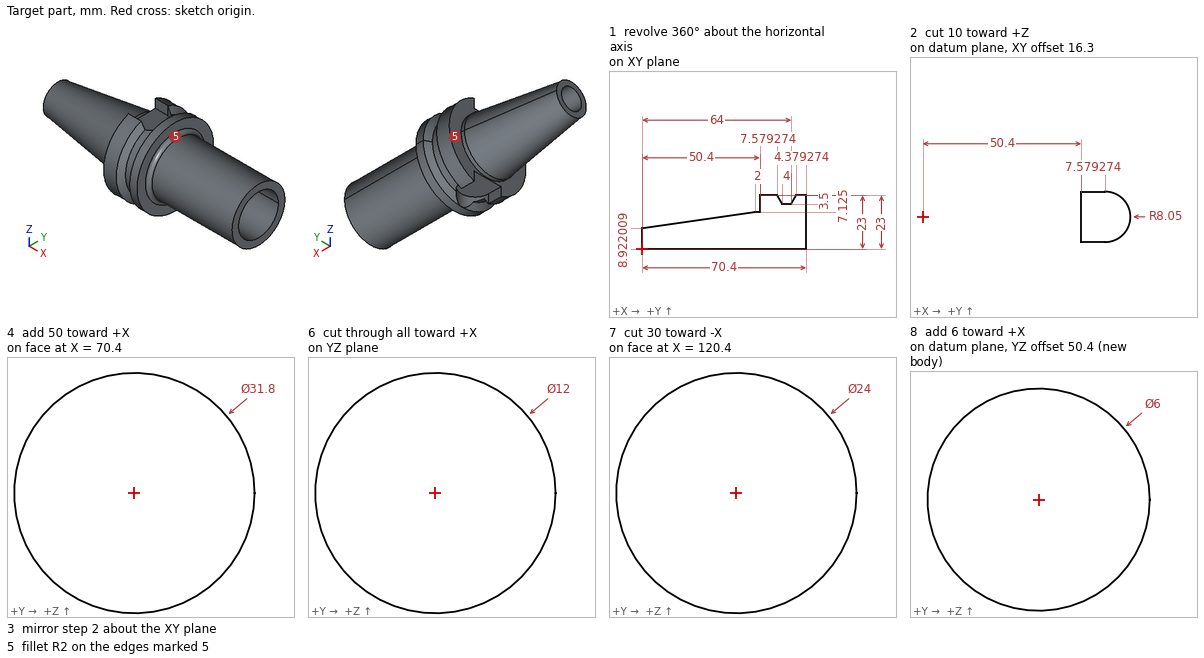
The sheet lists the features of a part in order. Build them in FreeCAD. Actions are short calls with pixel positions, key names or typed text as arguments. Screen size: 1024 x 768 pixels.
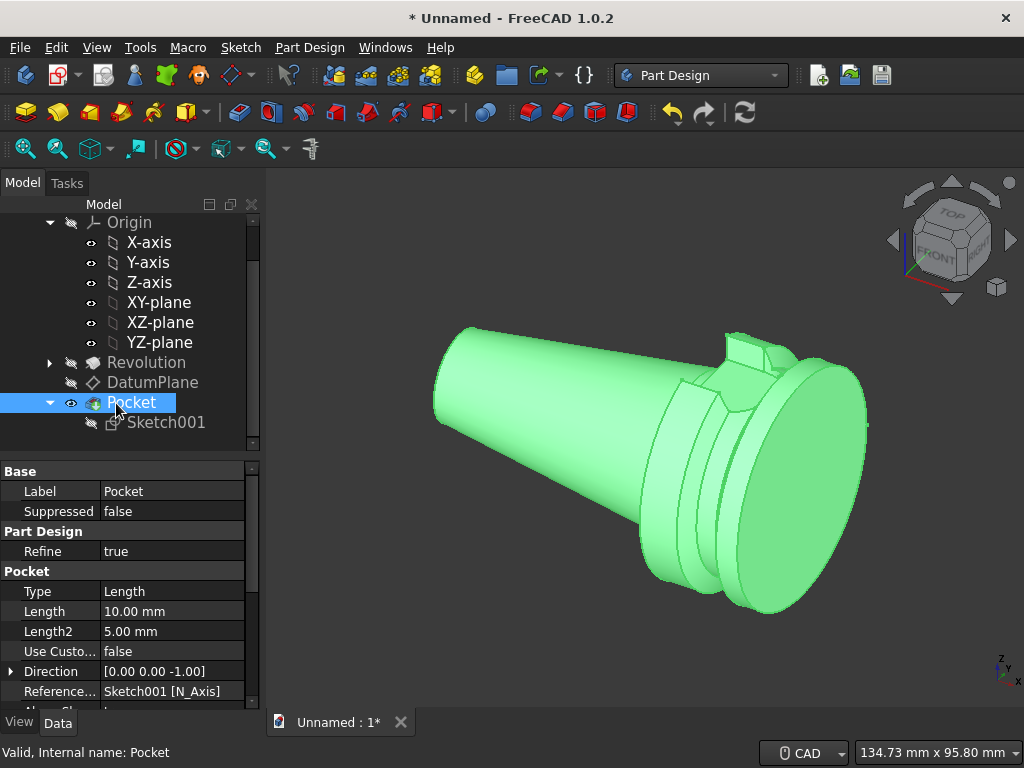
click(334, 76)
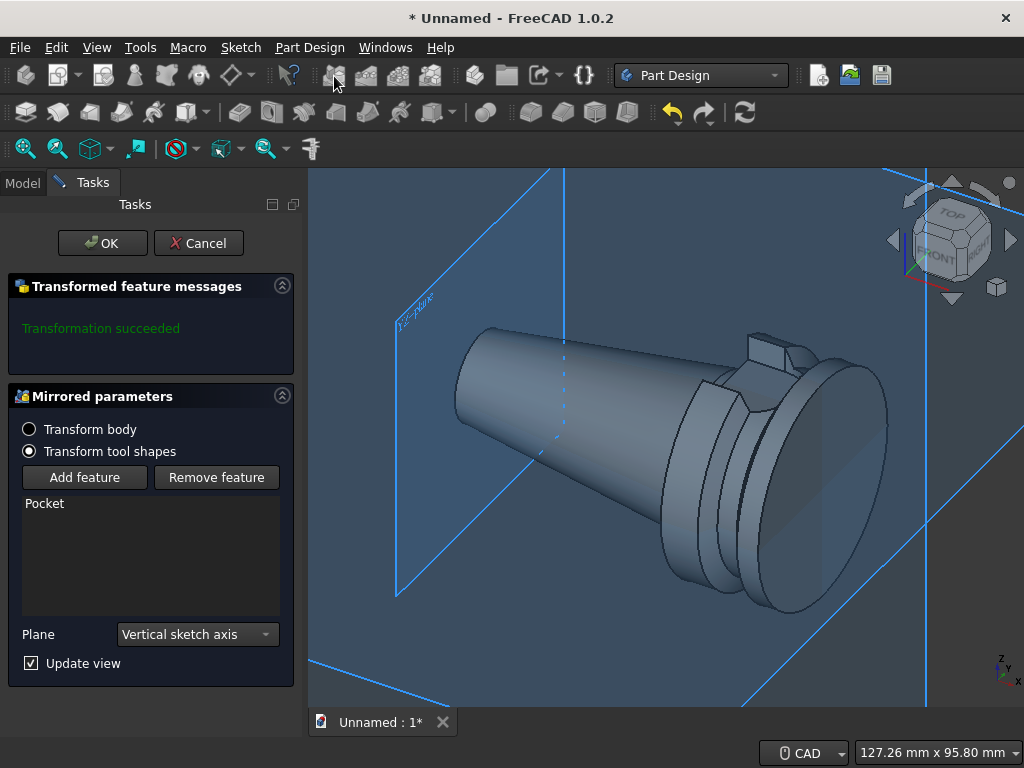
click(198, 634)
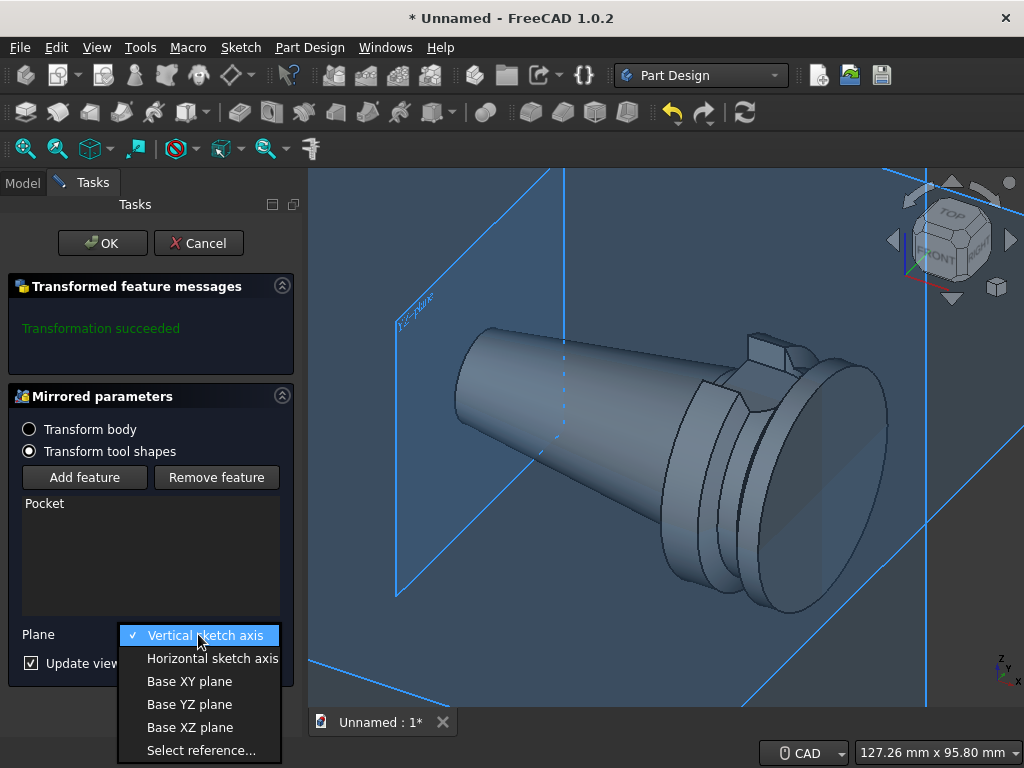
click(198, 682)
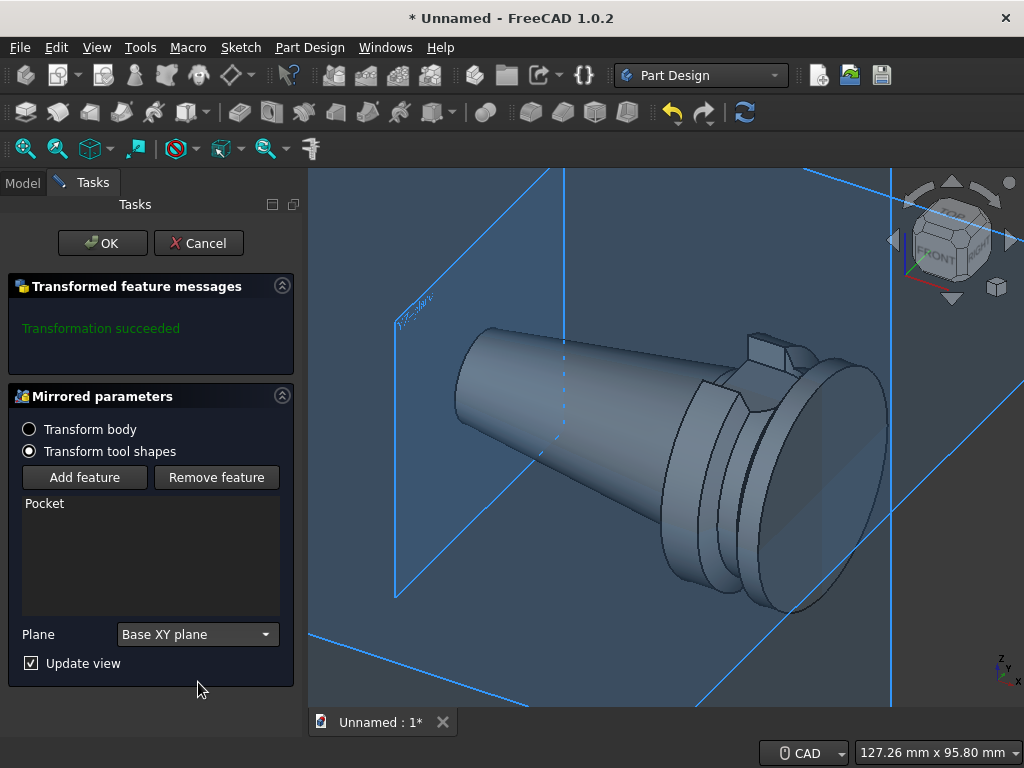
click(103, 243)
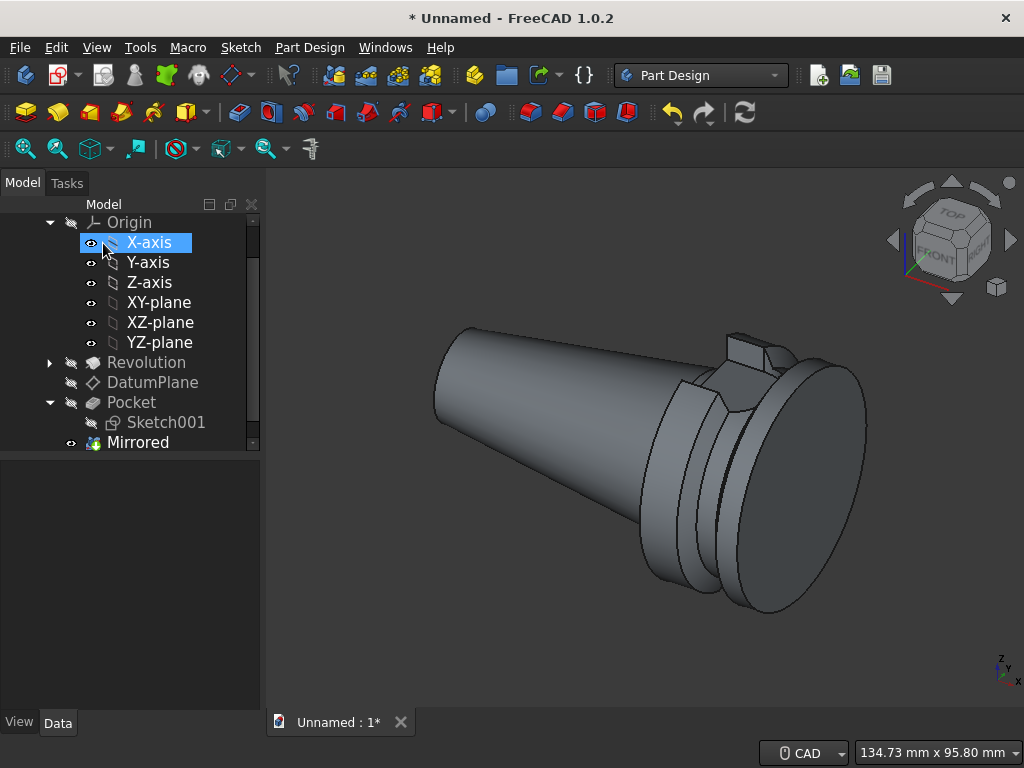
click(802, 488)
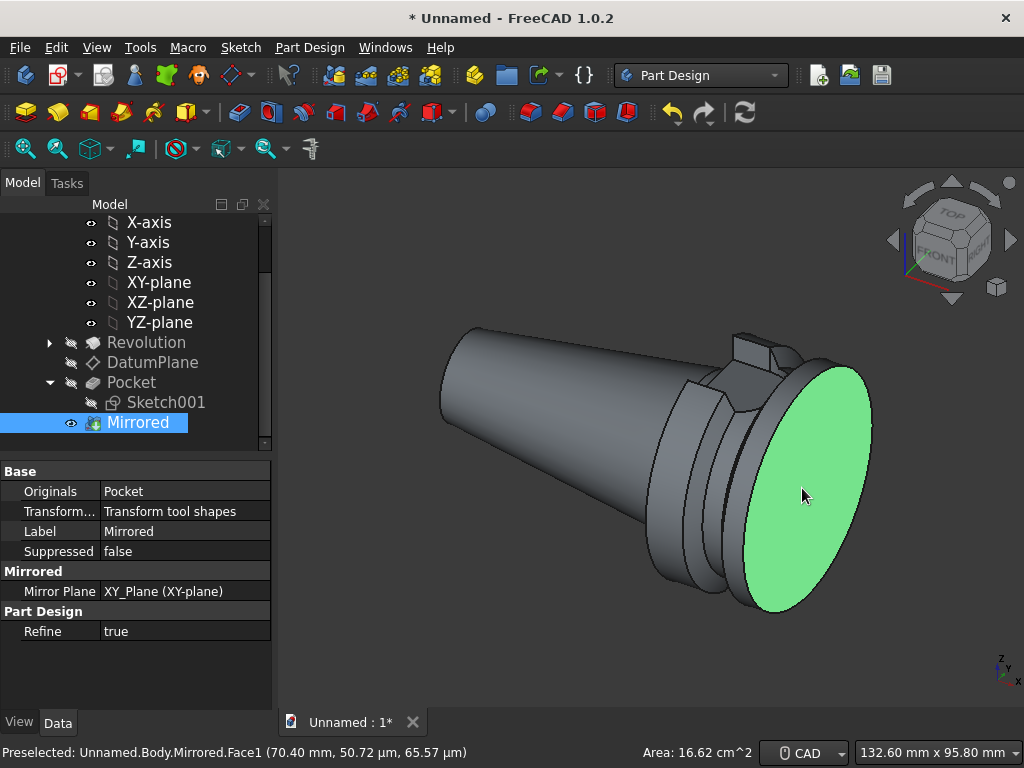
click(58, 76)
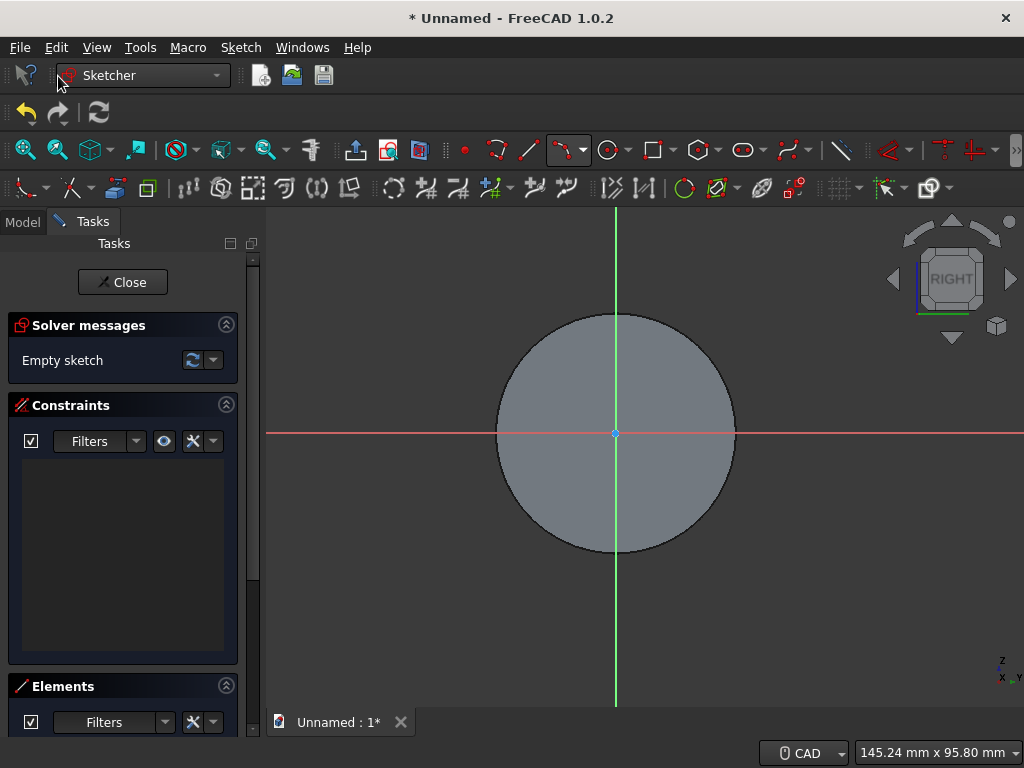
scroll(664, 405, up, 3)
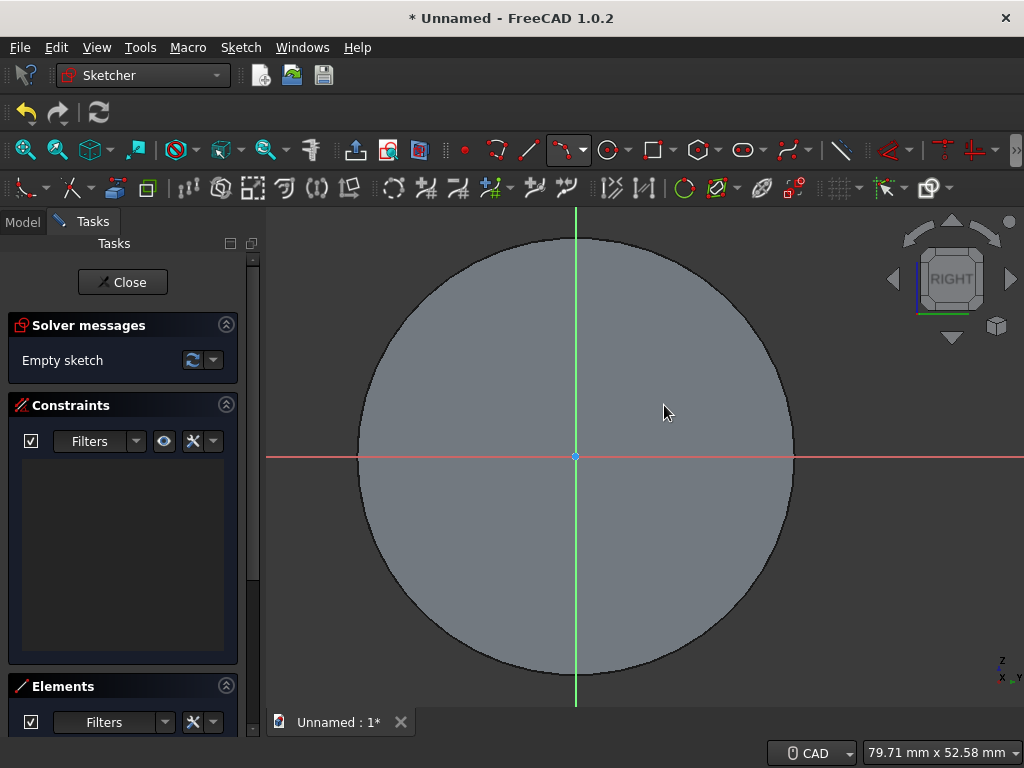
key(g)
key(c)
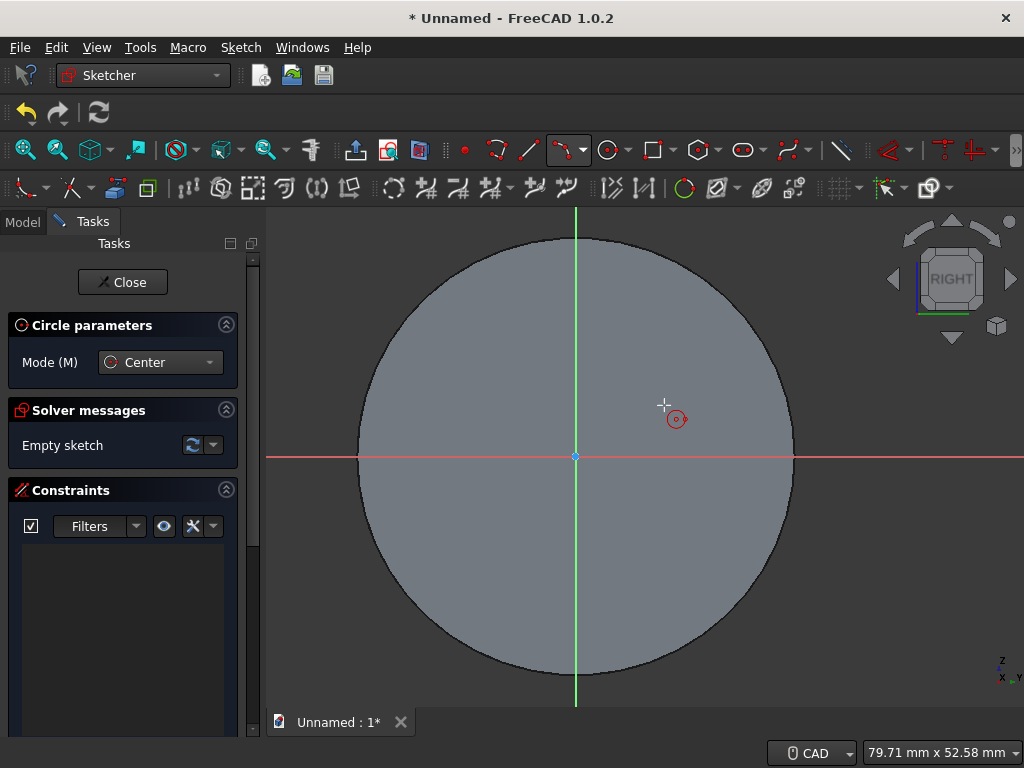
click(576, 457)
move(683, 350)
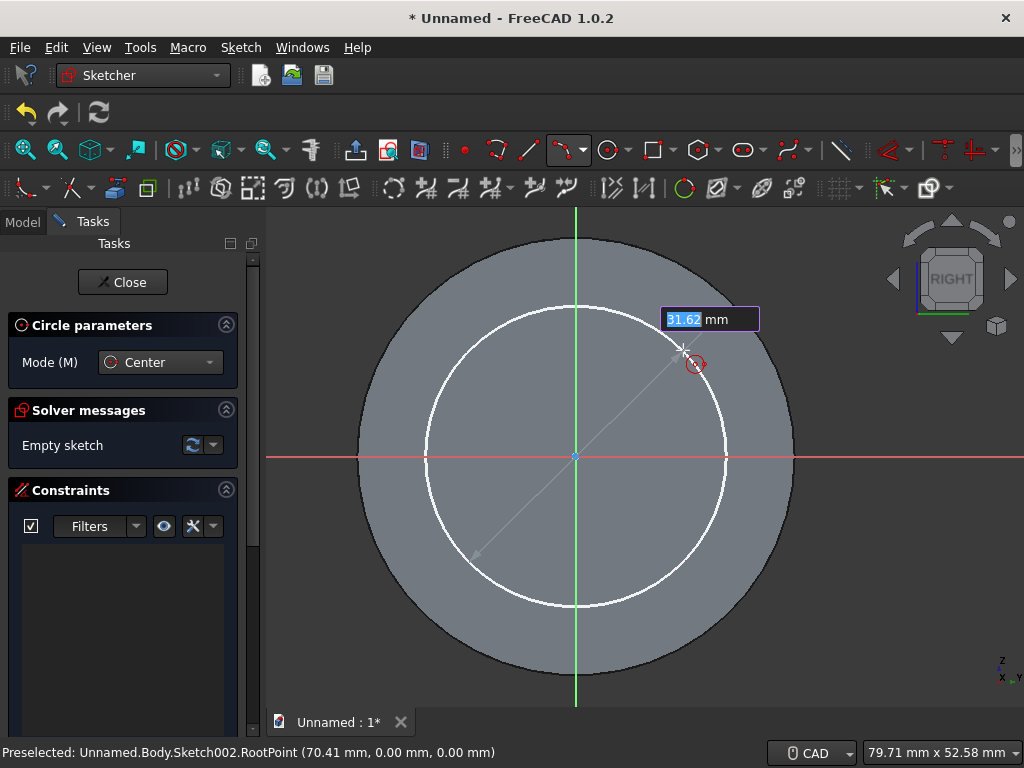
text(31.8)
key(Return)
key(Escape)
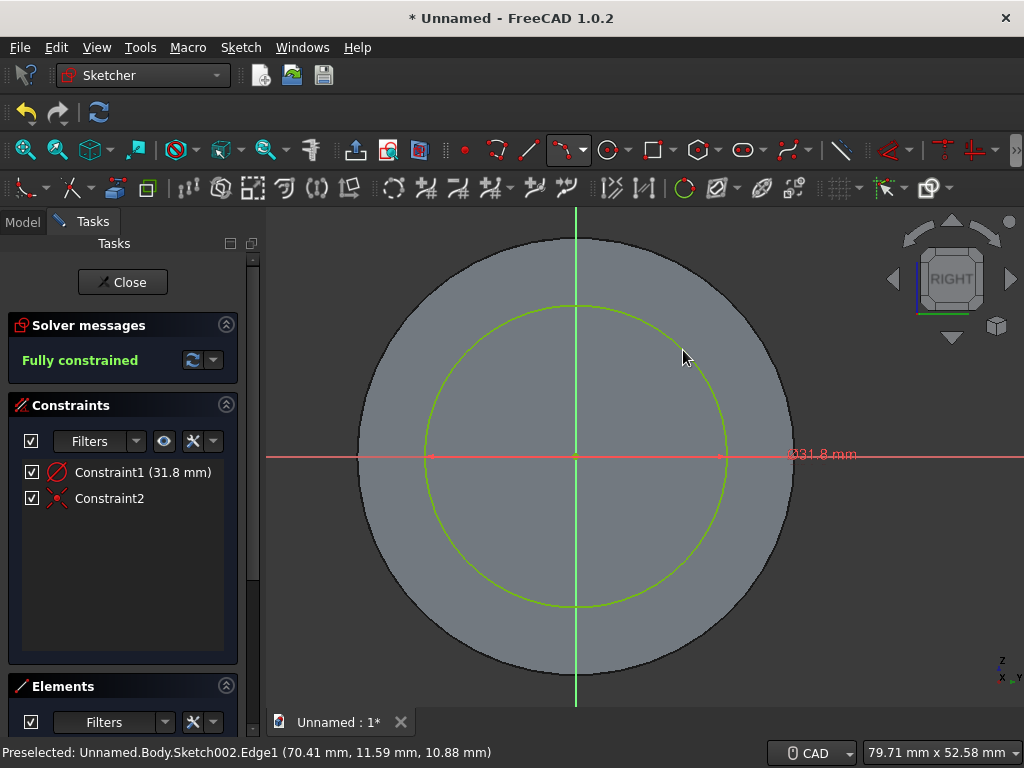
click(123, 282)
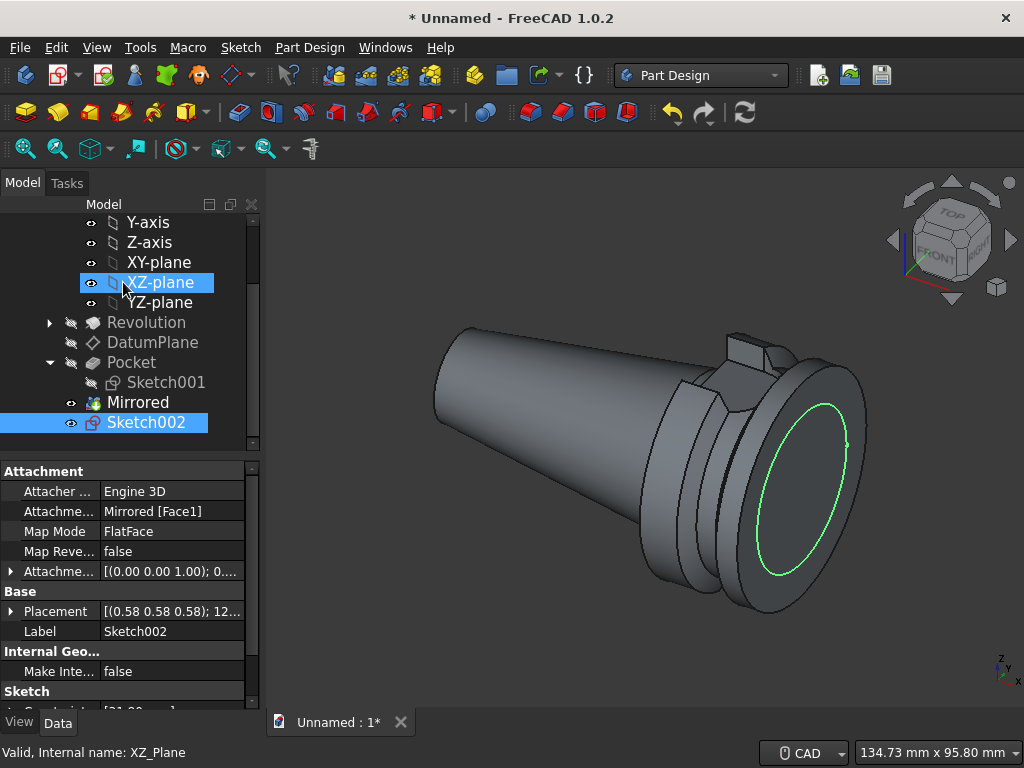
click(26, 112)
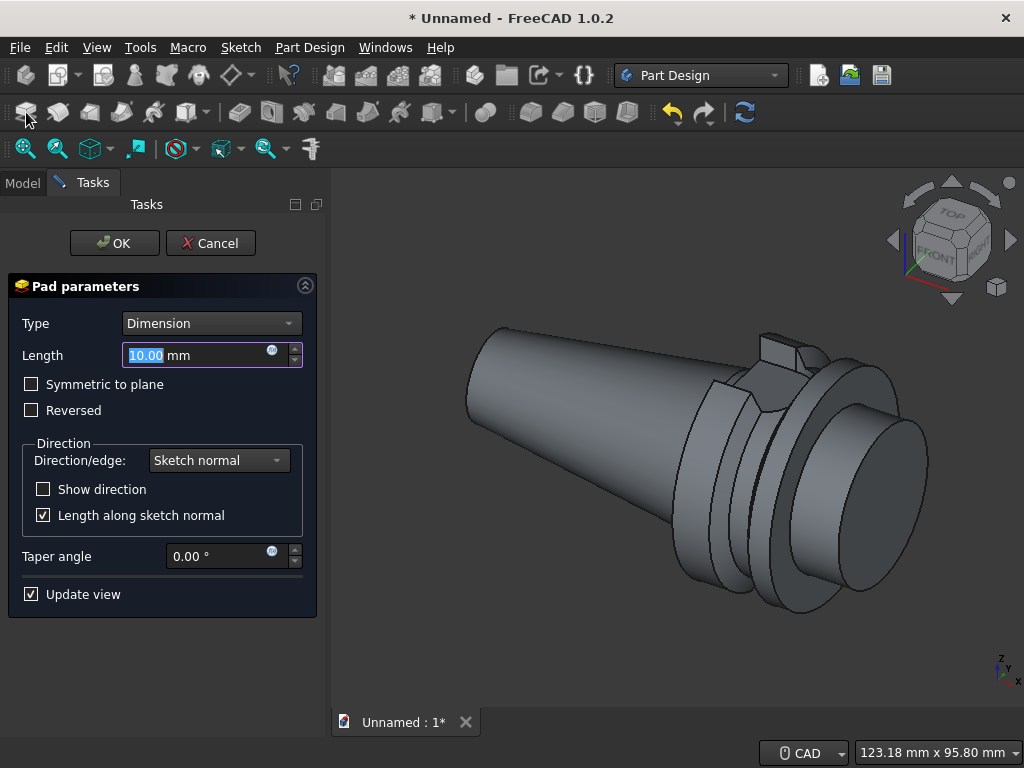
text(50)
key(Tab)